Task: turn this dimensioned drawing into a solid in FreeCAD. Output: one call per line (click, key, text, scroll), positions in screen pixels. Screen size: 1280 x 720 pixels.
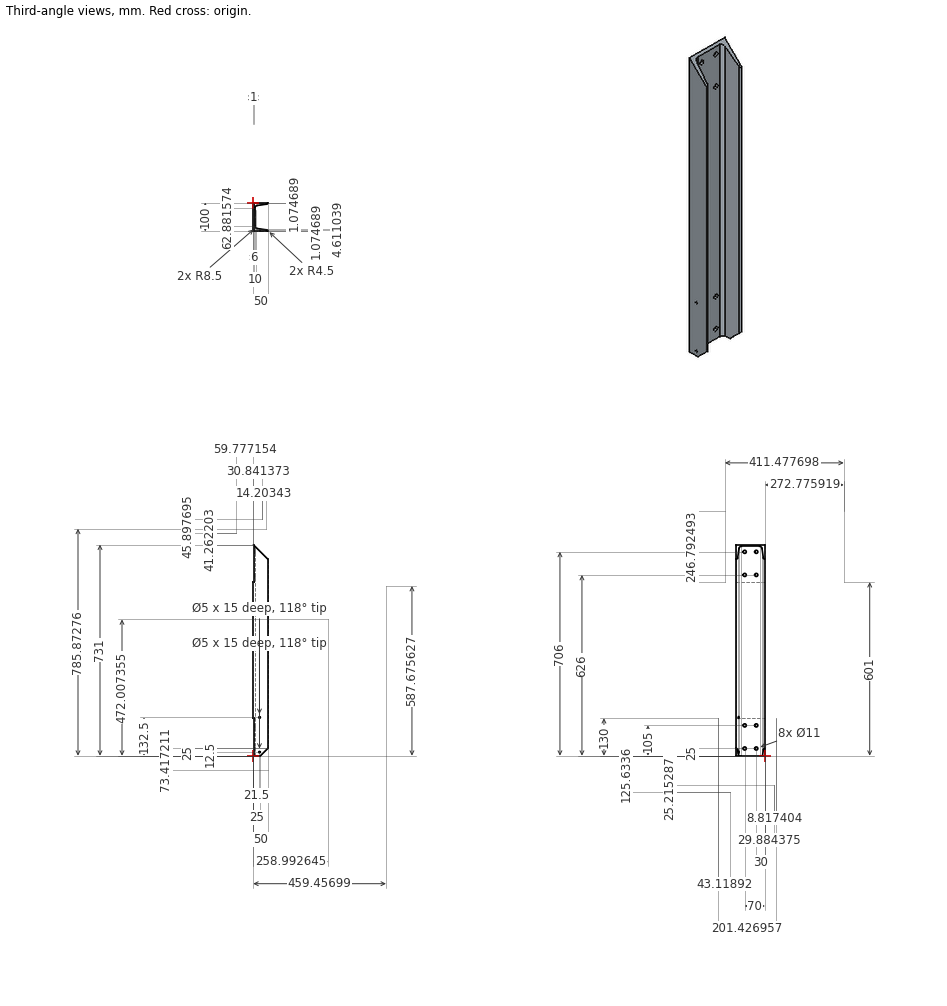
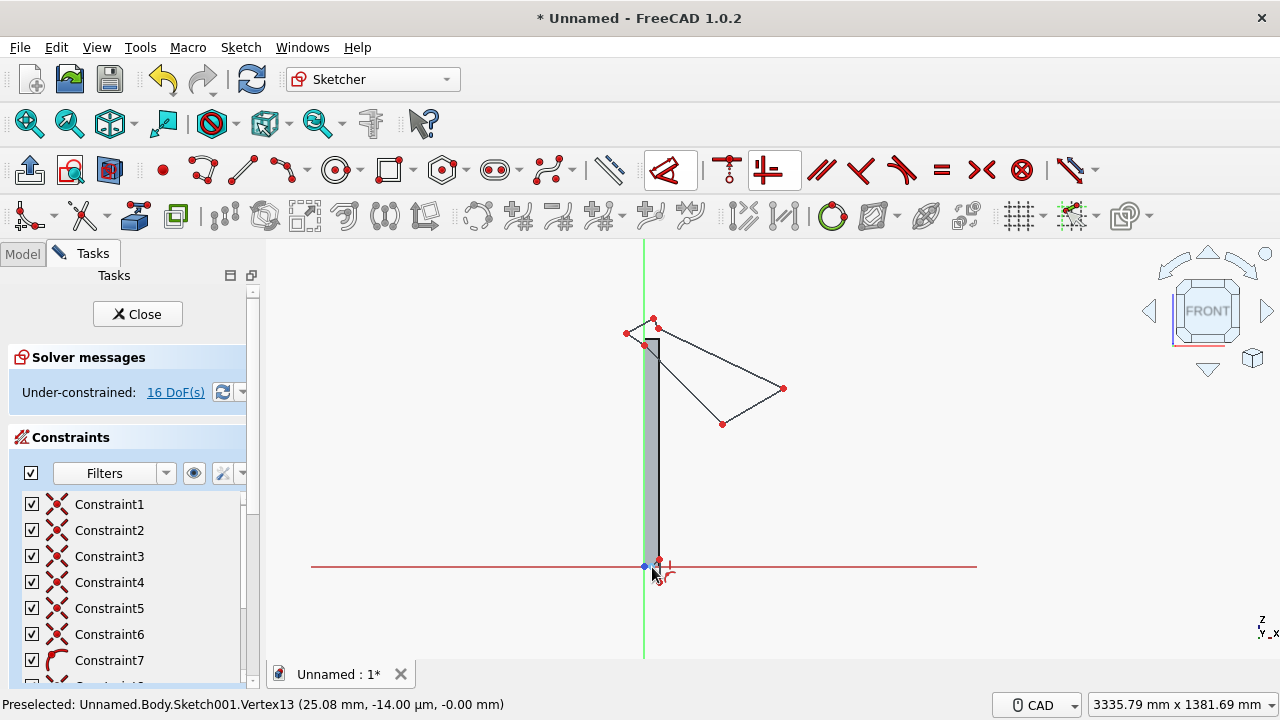
click(645, 345)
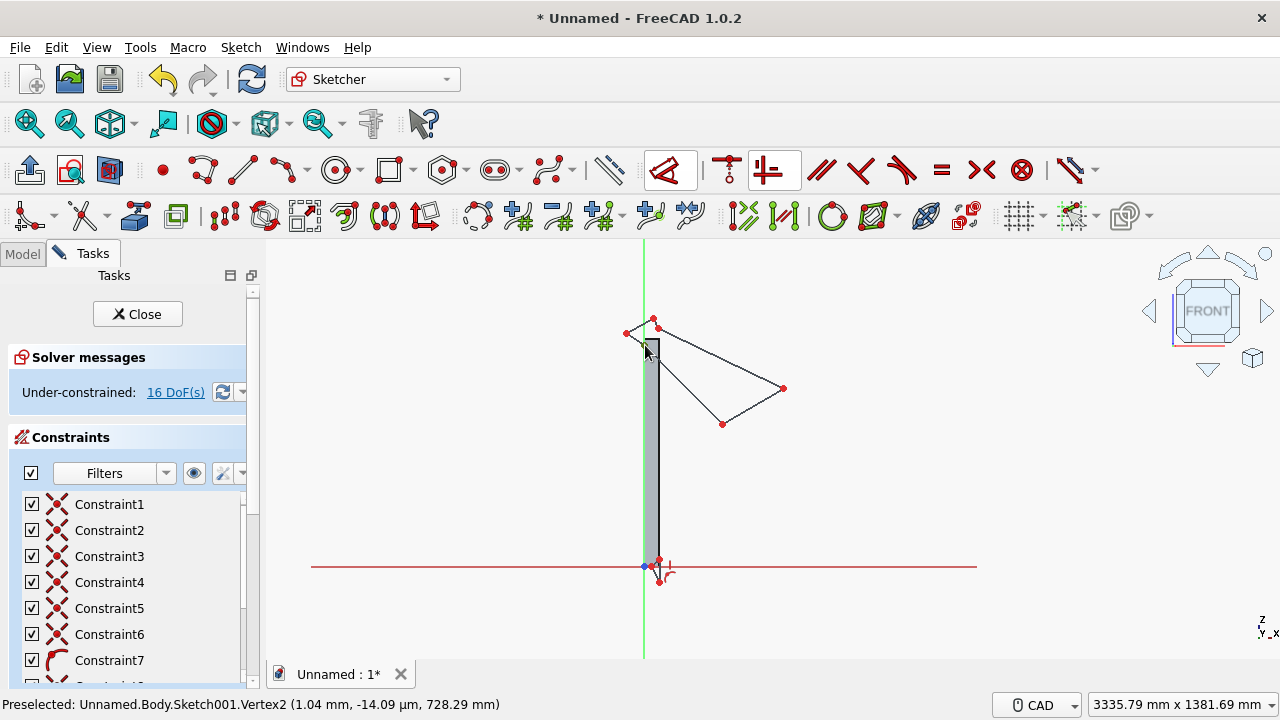
click(644, 527)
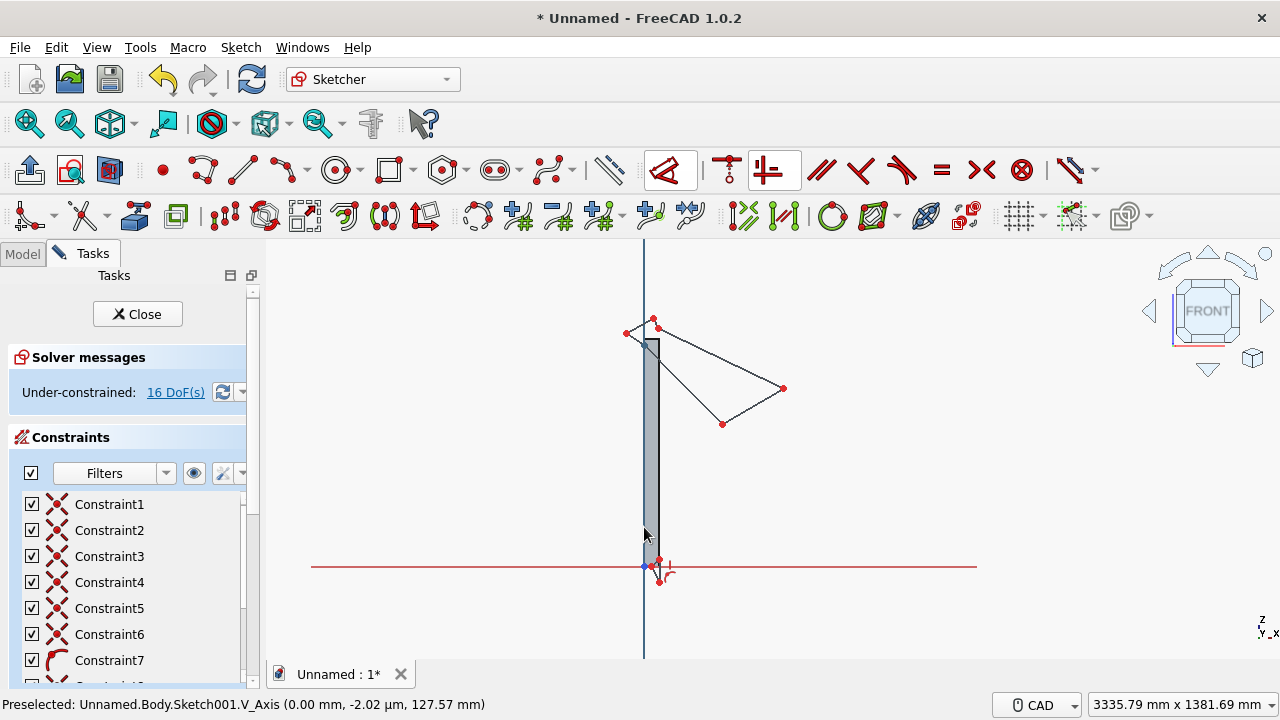
key(c)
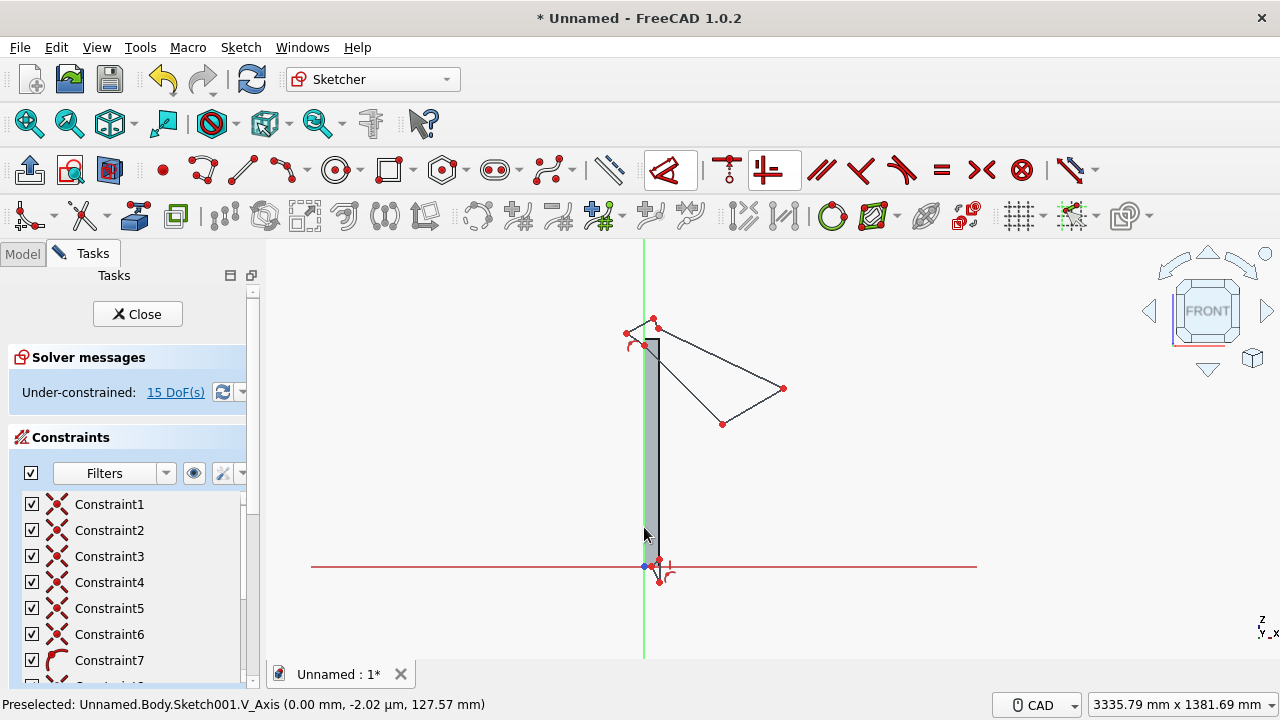
key(d)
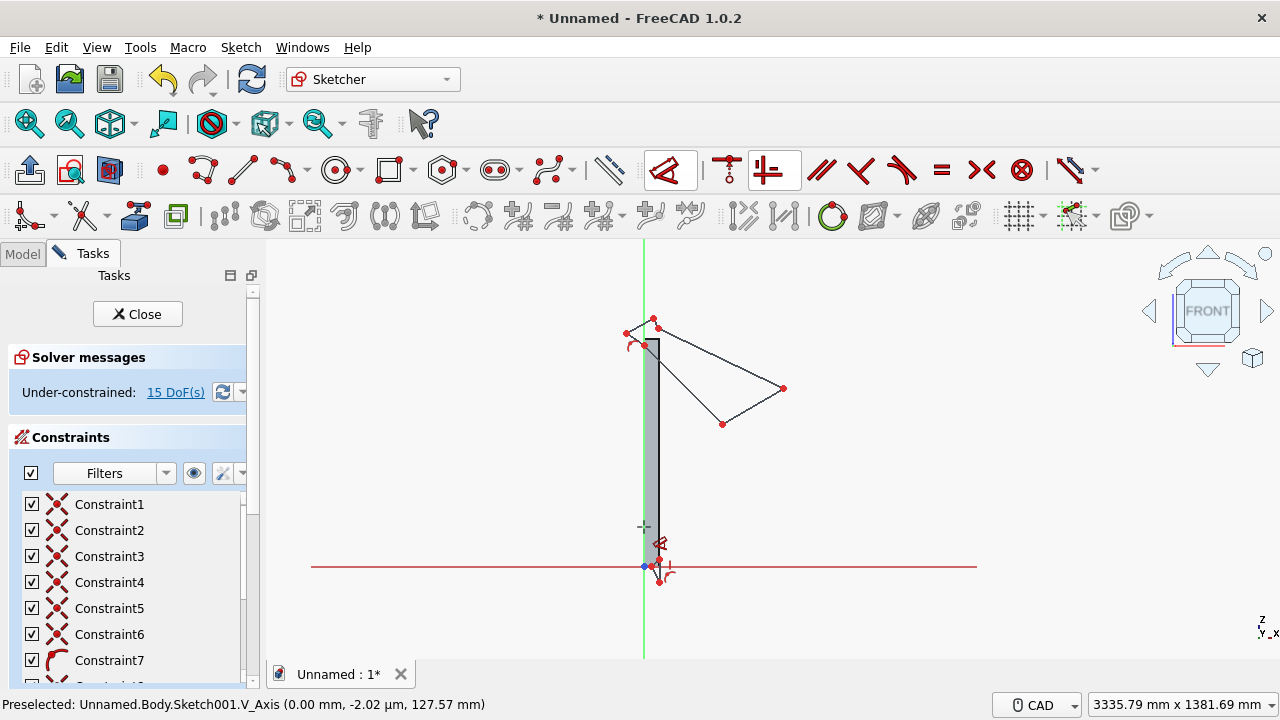
scroll(652, 567, up, 9)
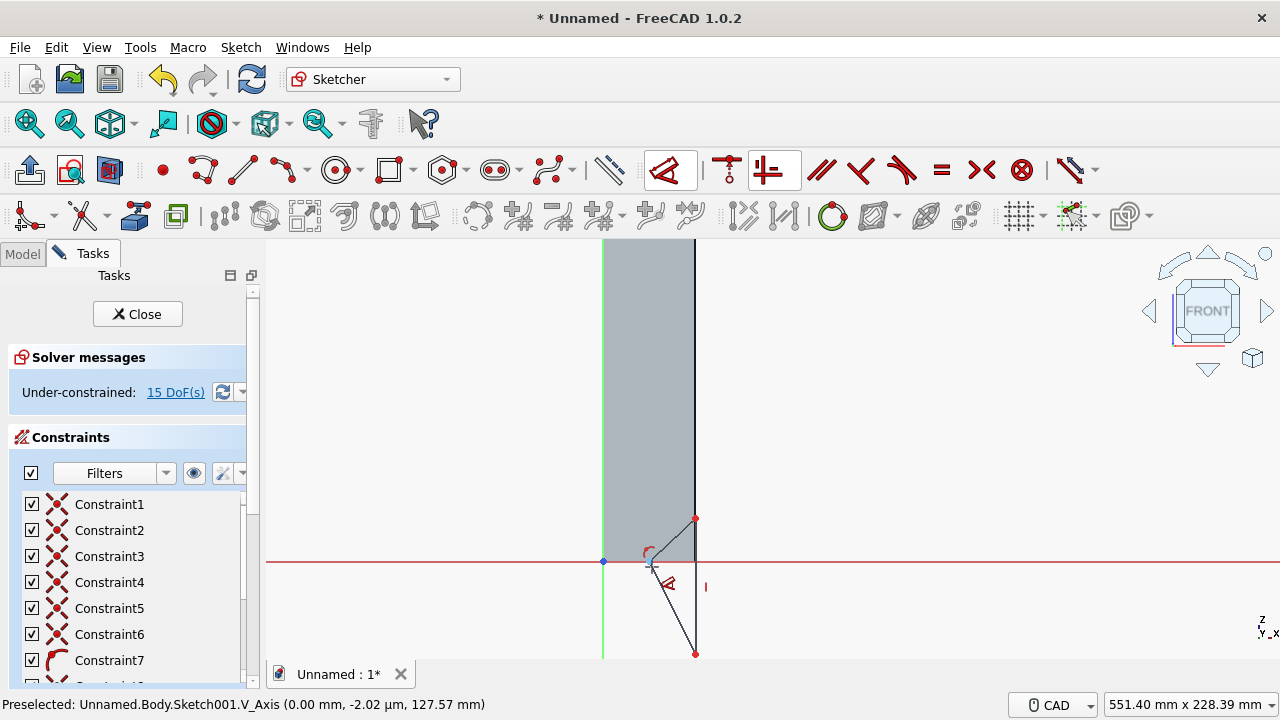
click(650, 562)
click(626, 596)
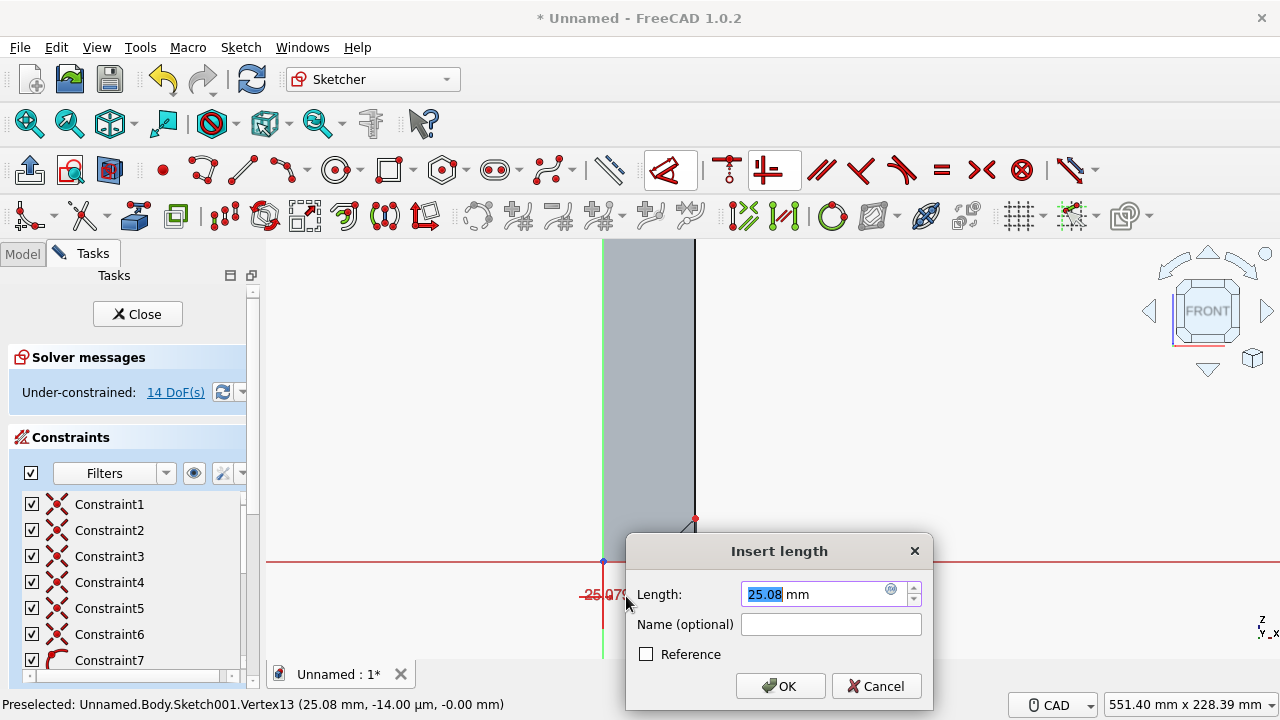
text(25)
key(Return)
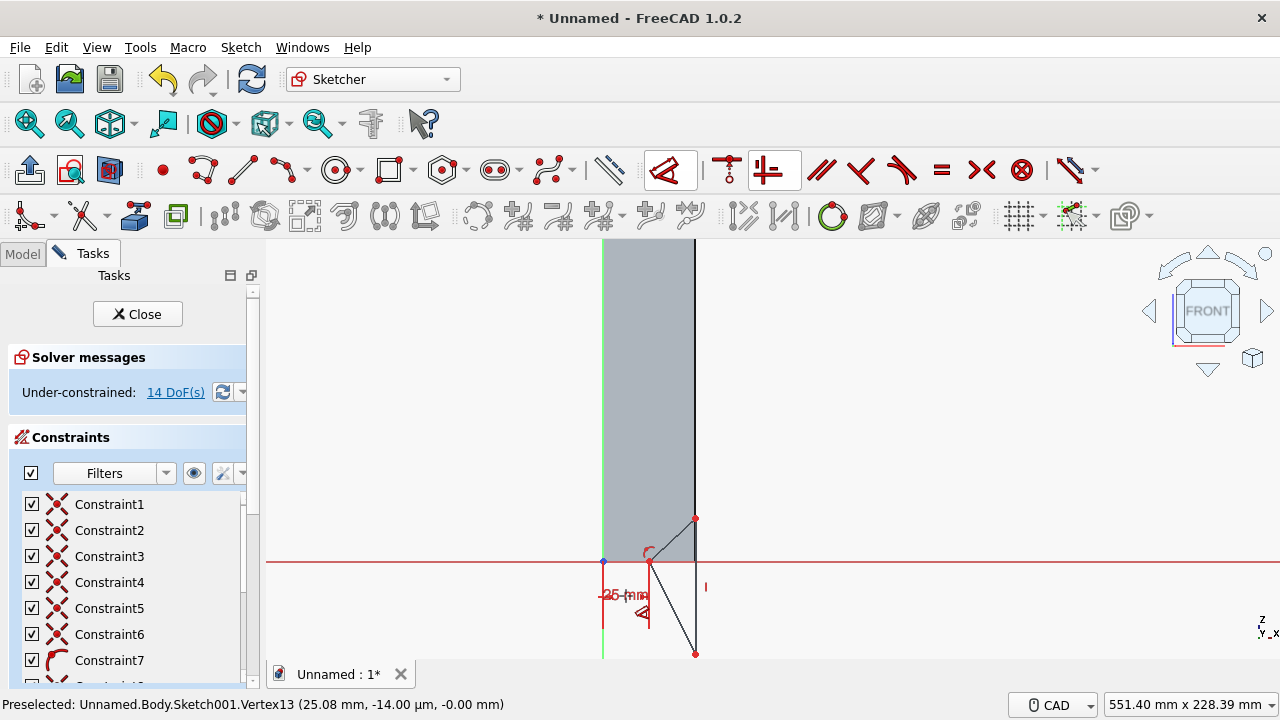
click(696, 519)
click(650, 485)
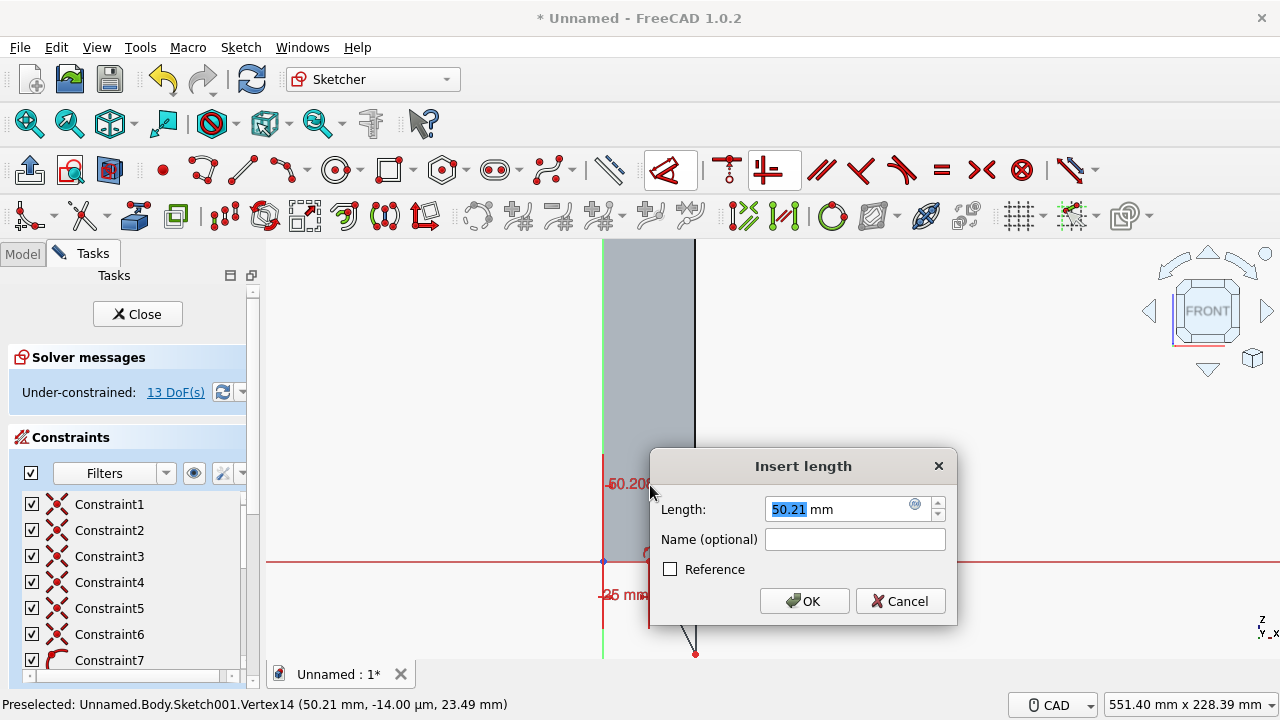
text(50)
key(Return)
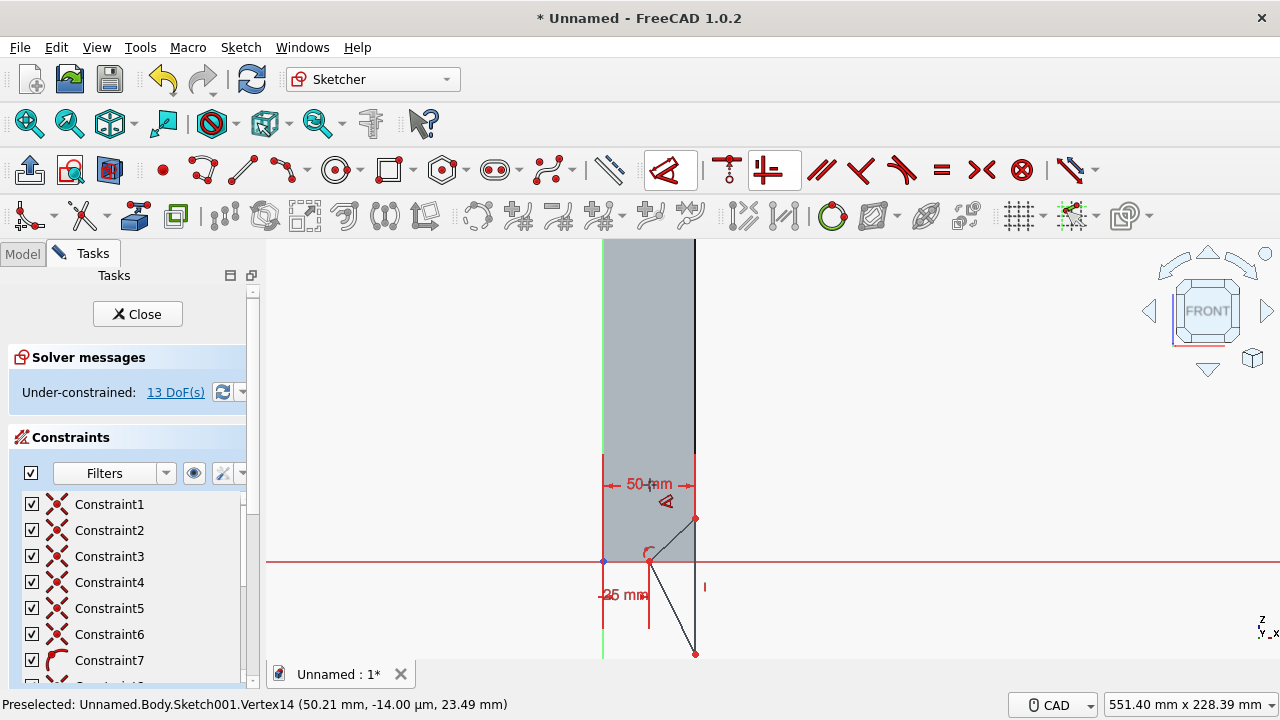
click(695, 519)
click(569, 540)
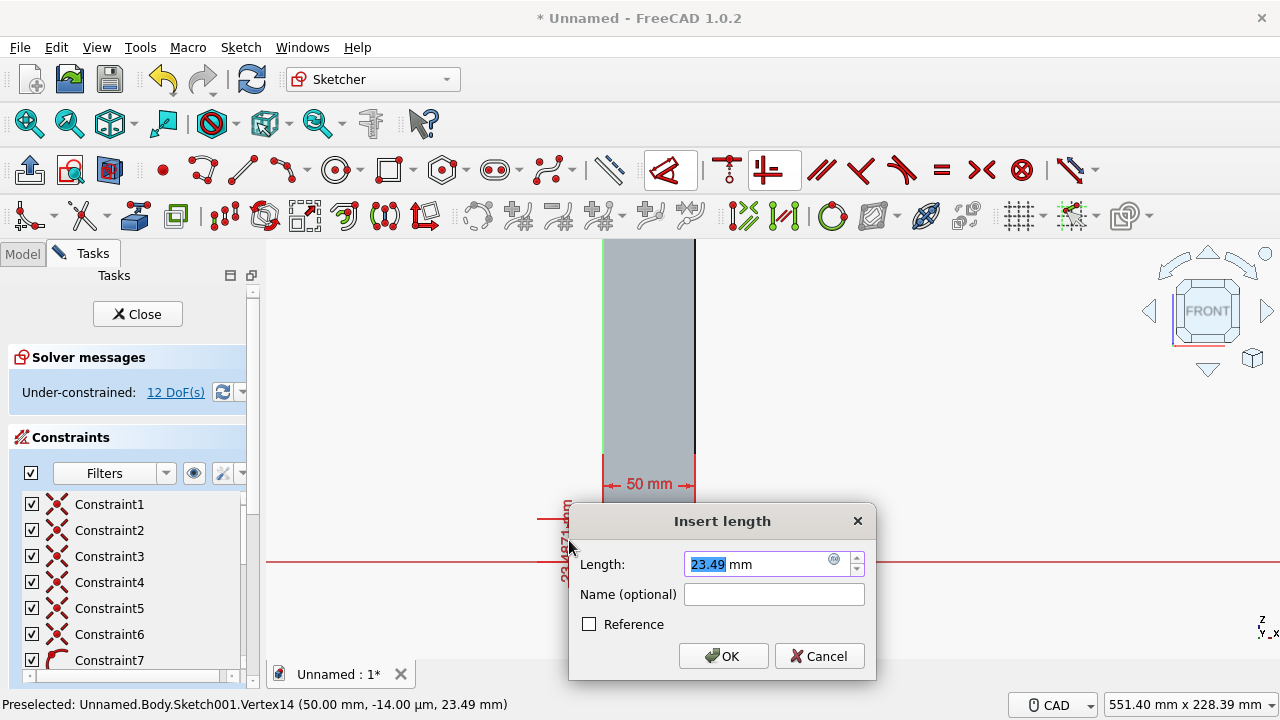
text(25)
key(Return)